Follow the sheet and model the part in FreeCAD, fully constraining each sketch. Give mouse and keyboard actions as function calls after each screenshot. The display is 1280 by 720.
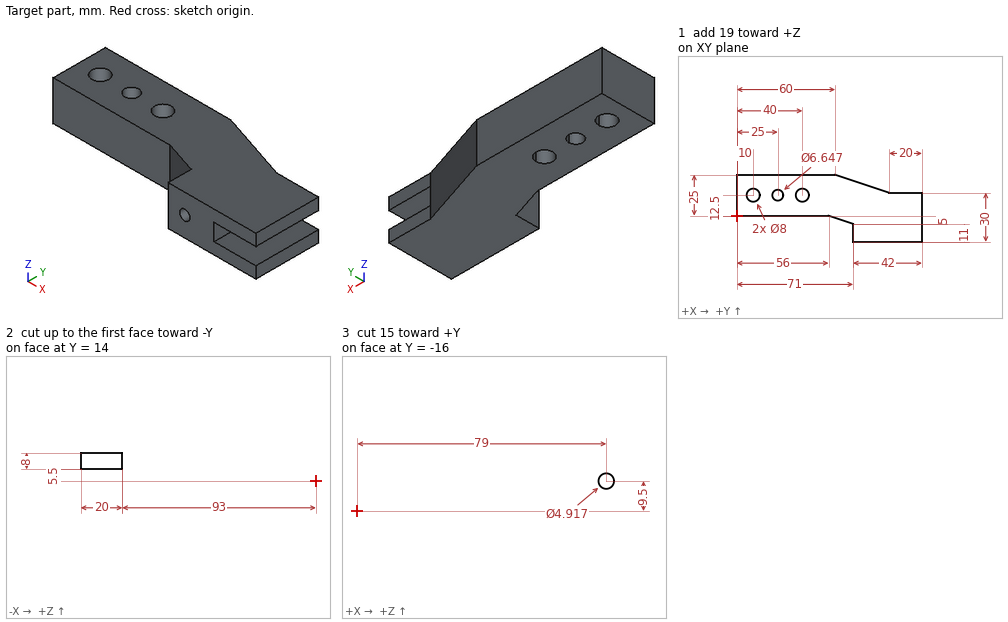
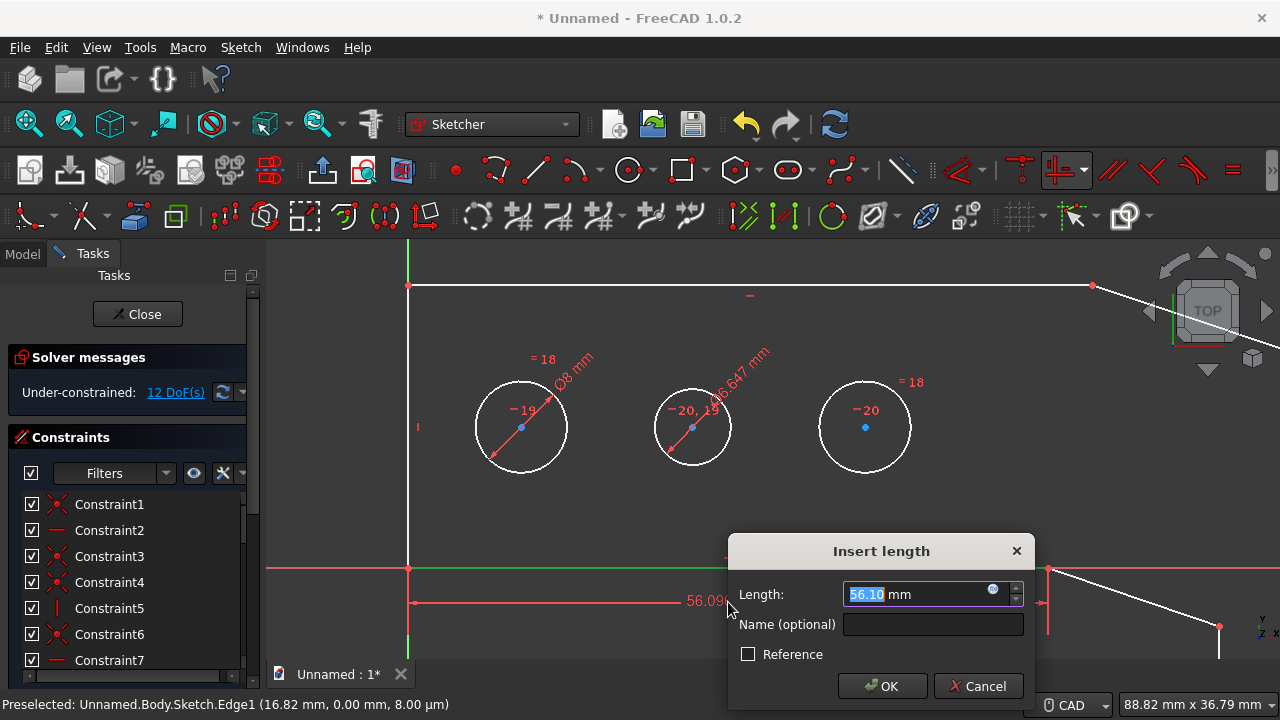
text(56)
key(Return)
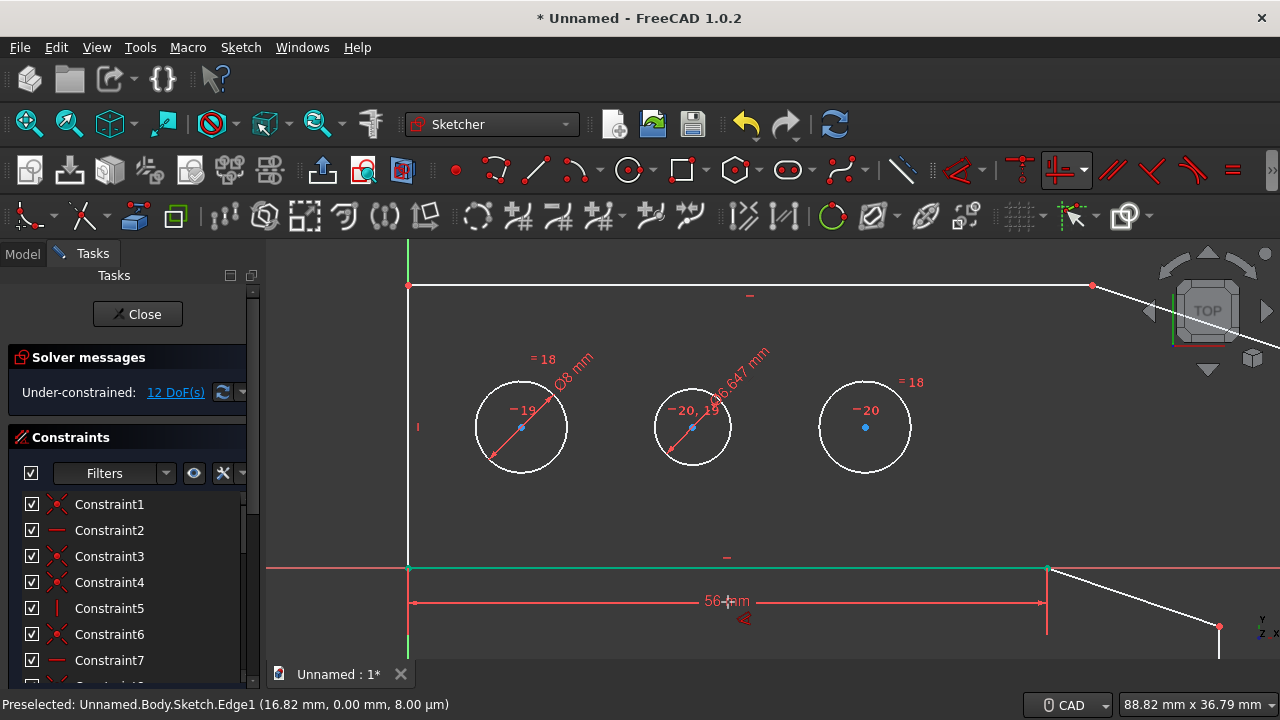
scroll(420, 394, down, 4)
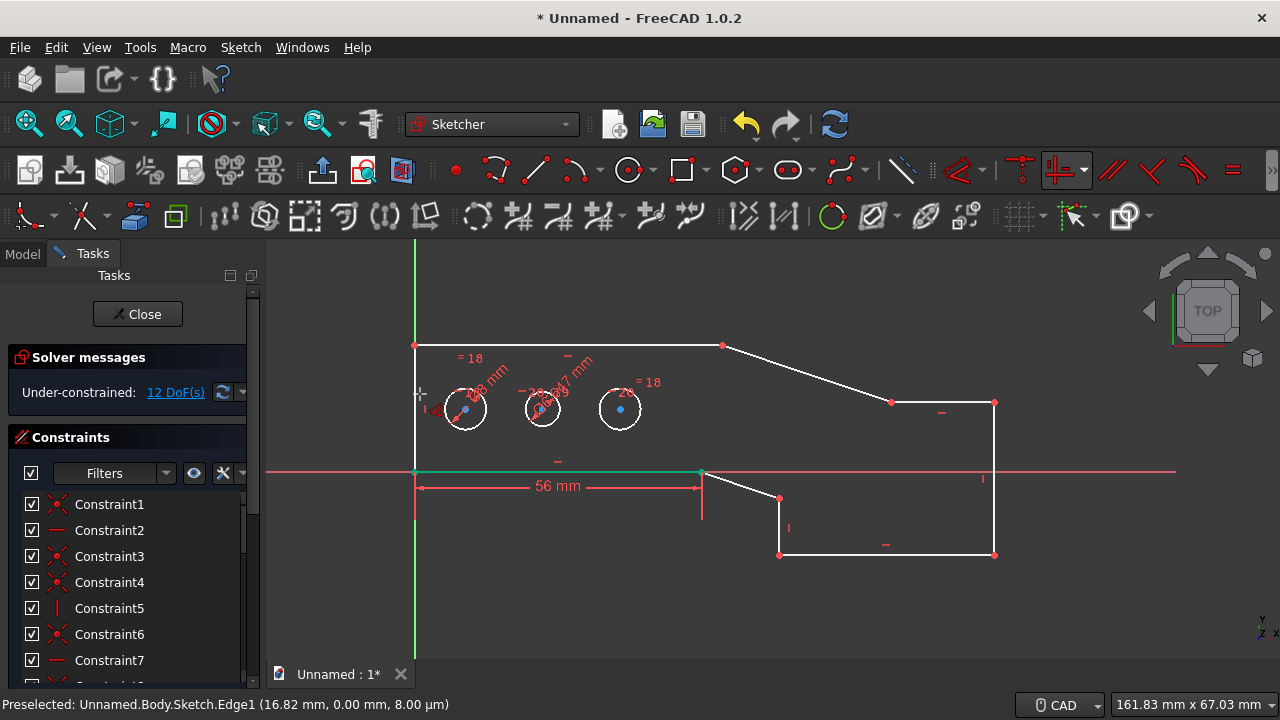
click(779, 516)
click(813, 527)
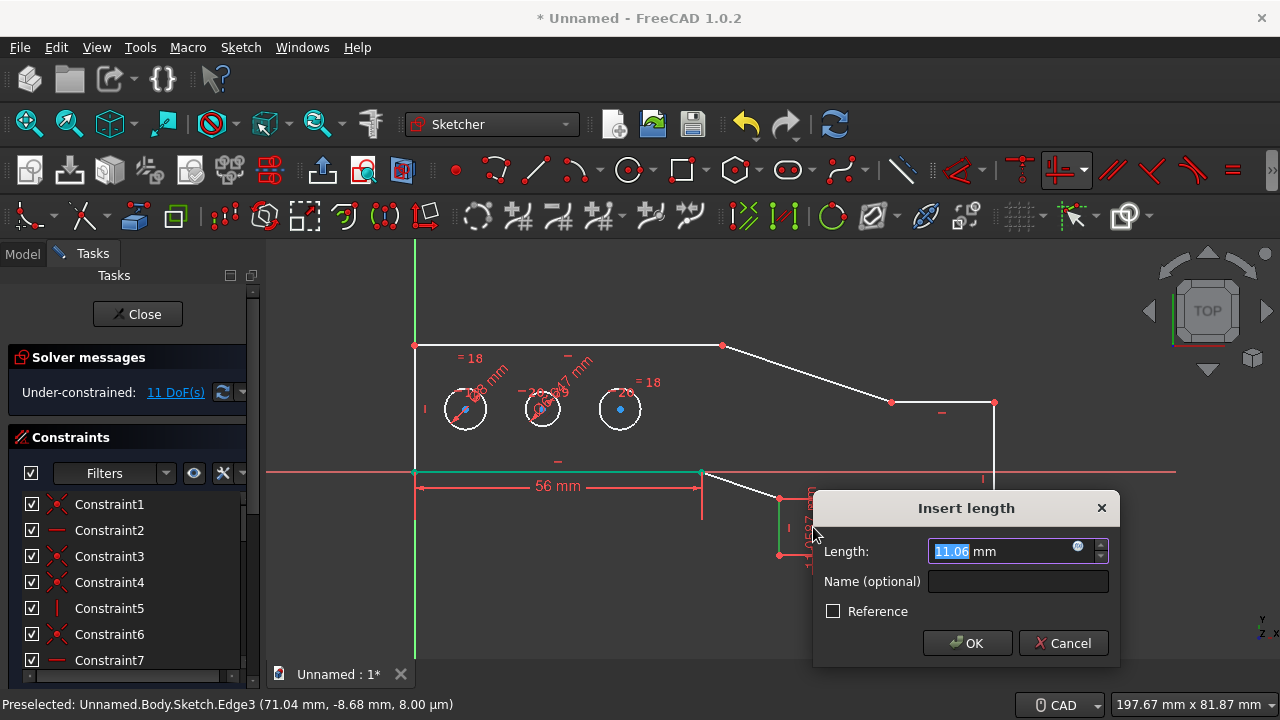
text(11)
key(Return)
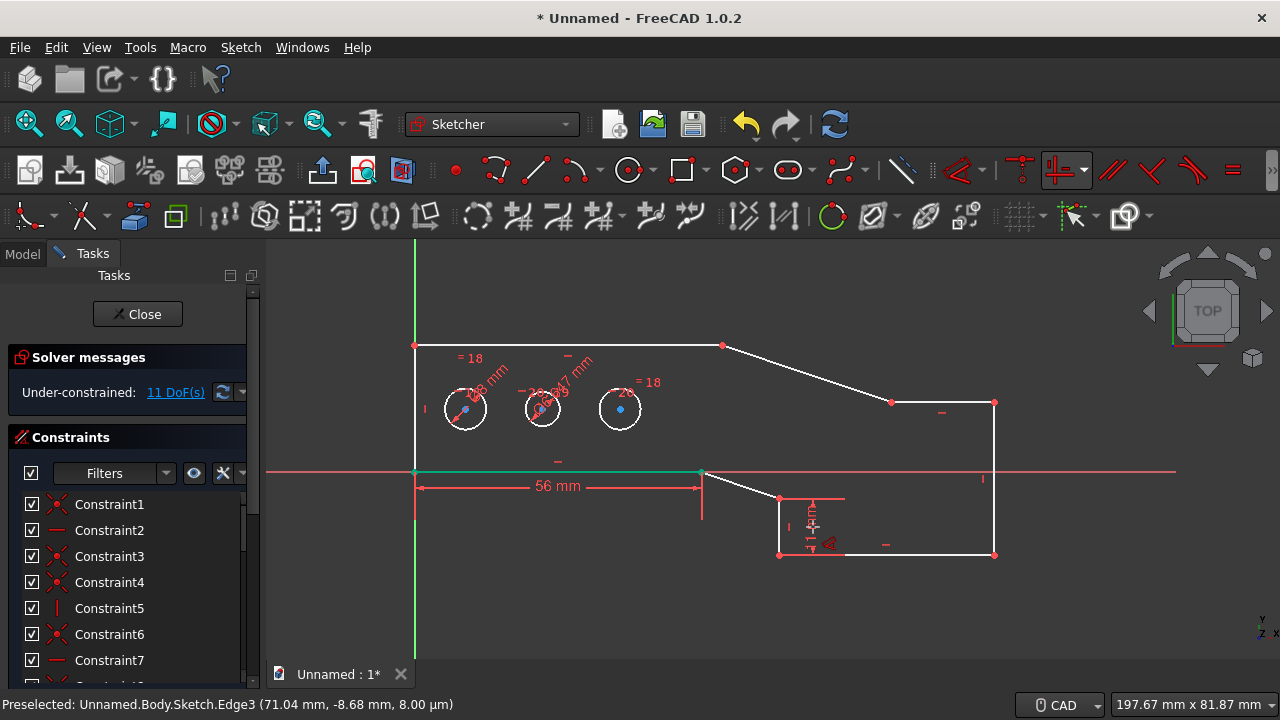
click(844, 555)
click(887, 589)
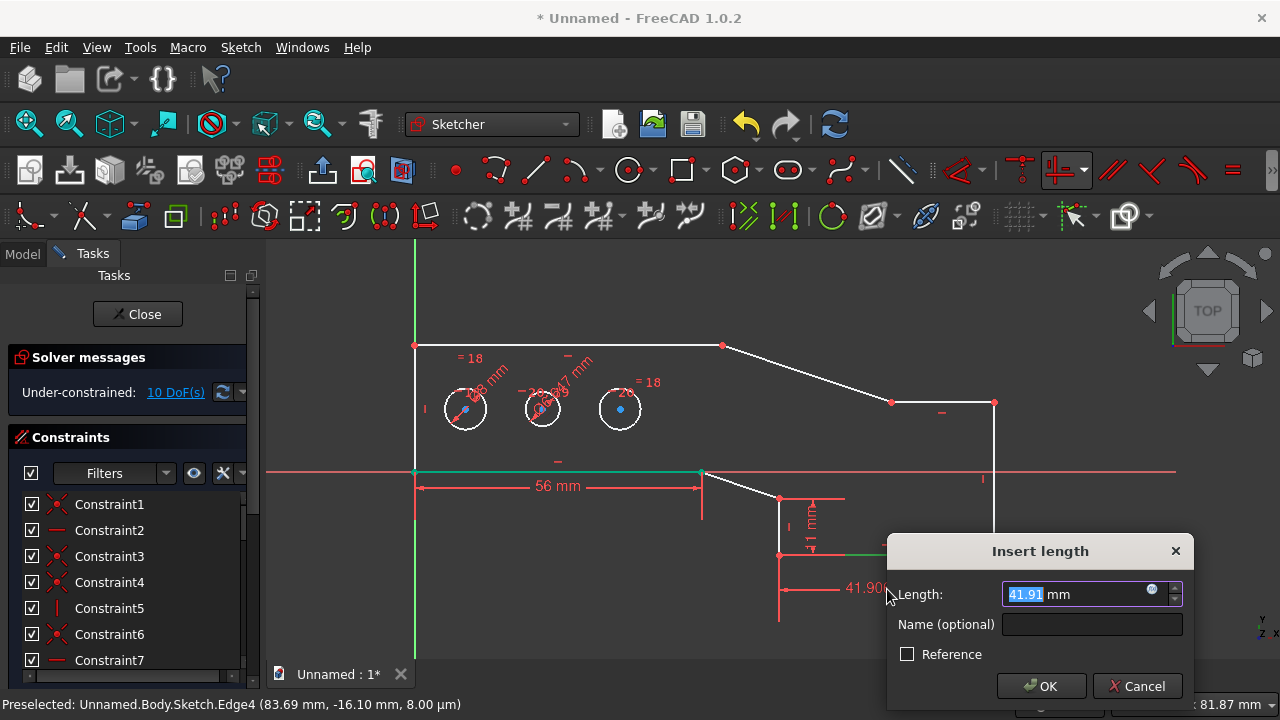
text(42)
key(Return)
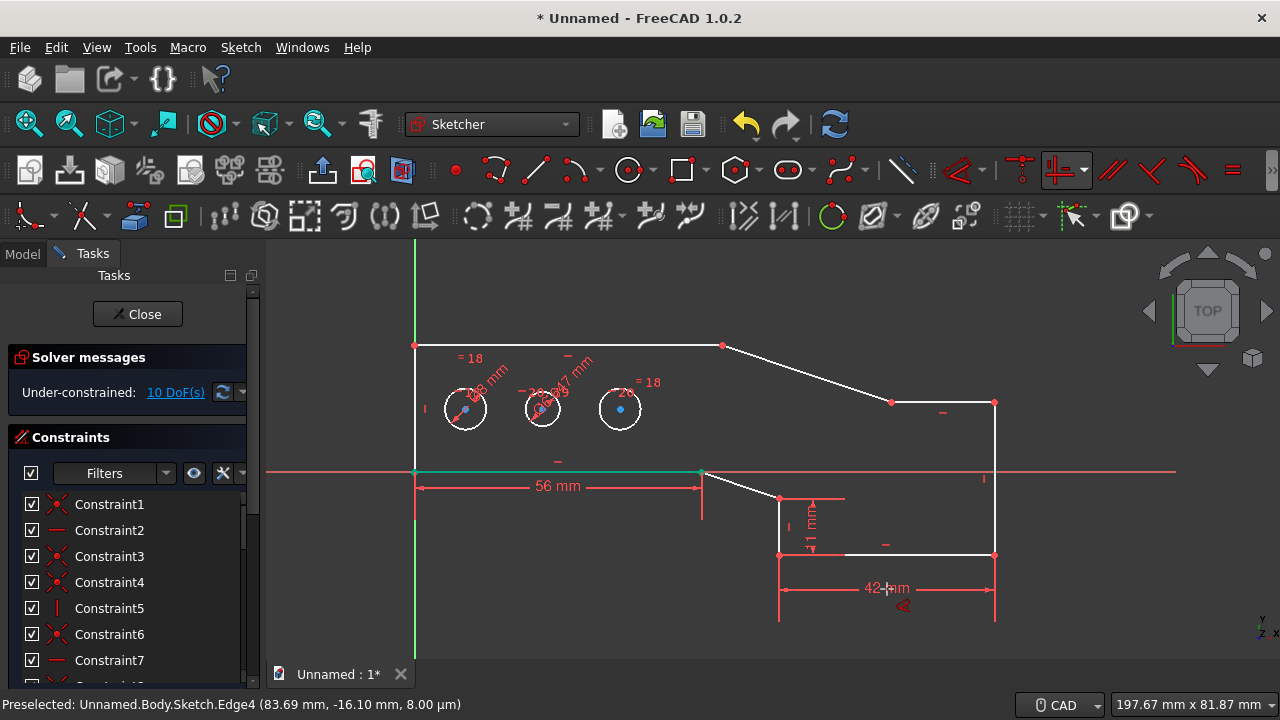
click(995, 509)
click(1029, 443)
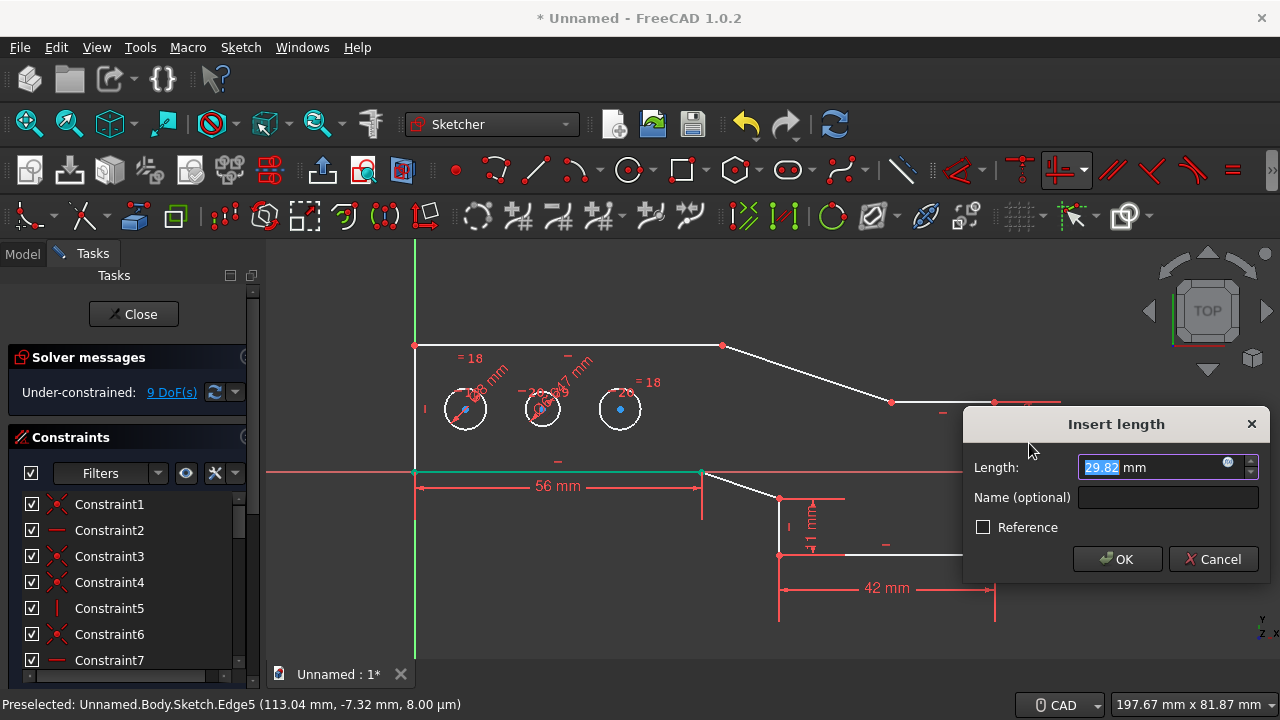
text(30)
key(Return)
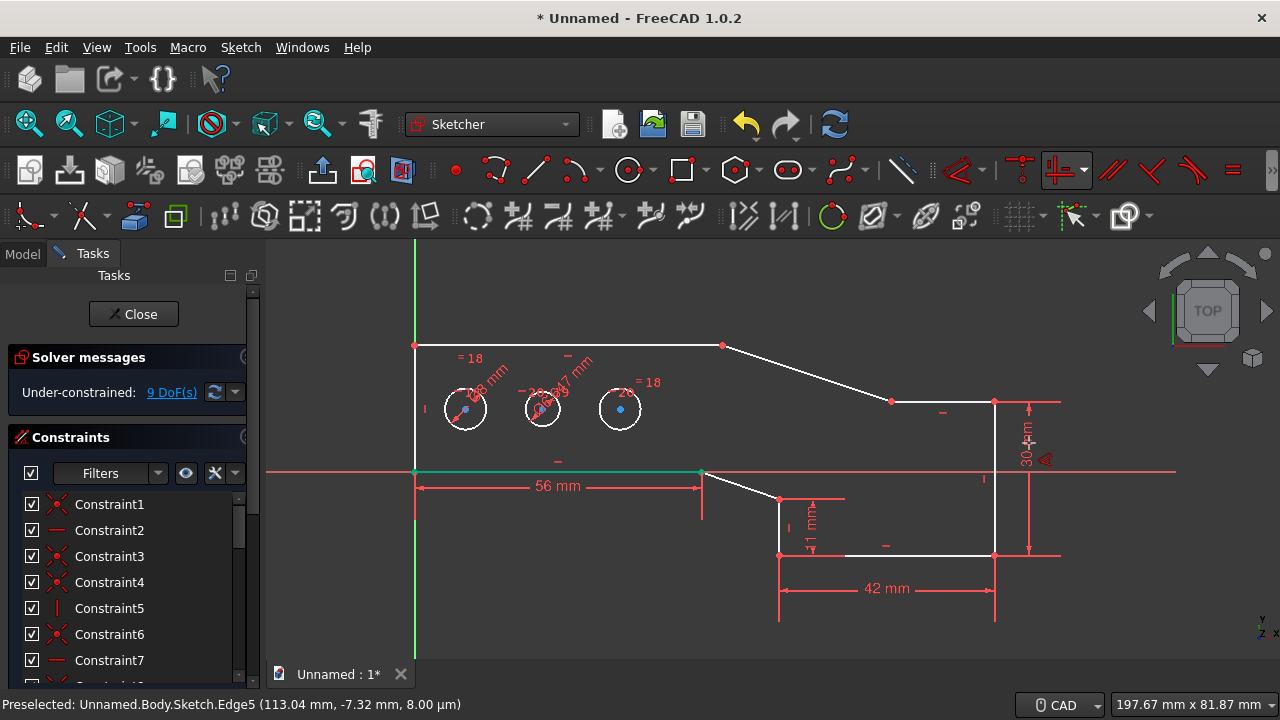
click(964, 402)
click(943, 368)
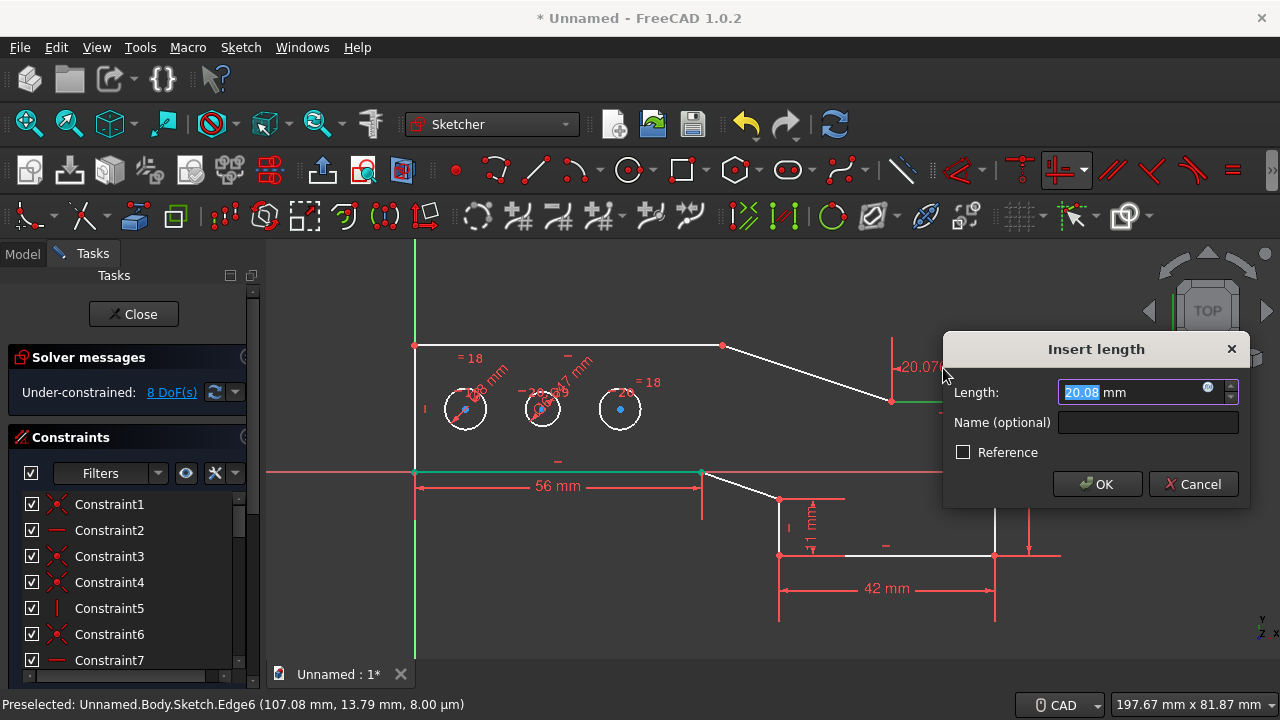
text(20)
key(Return)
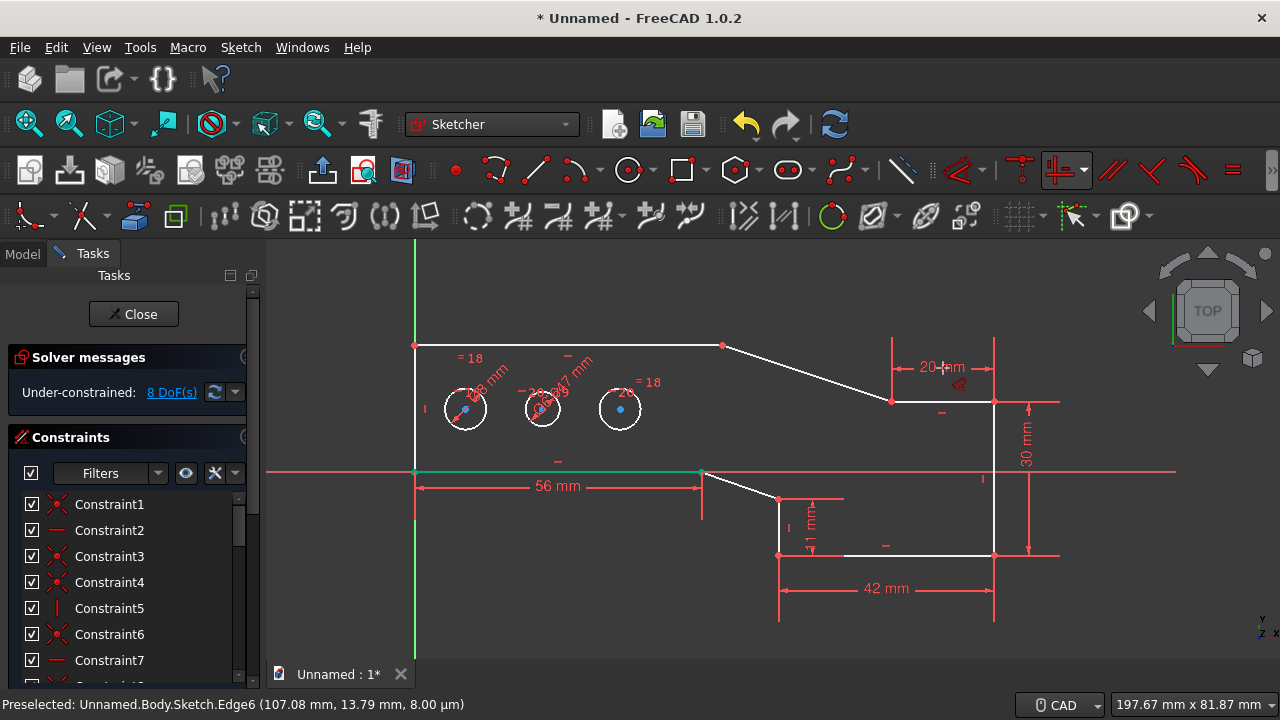
click(630, 345)
click(569, 311)